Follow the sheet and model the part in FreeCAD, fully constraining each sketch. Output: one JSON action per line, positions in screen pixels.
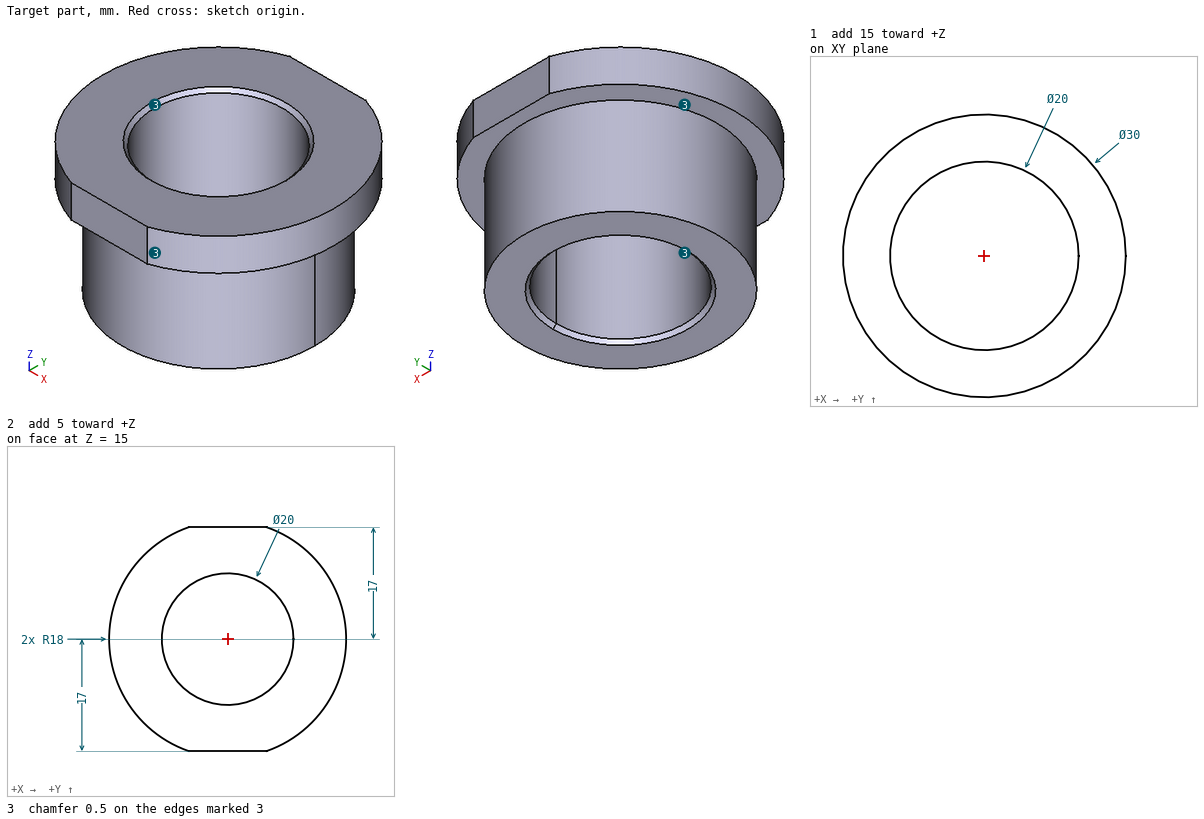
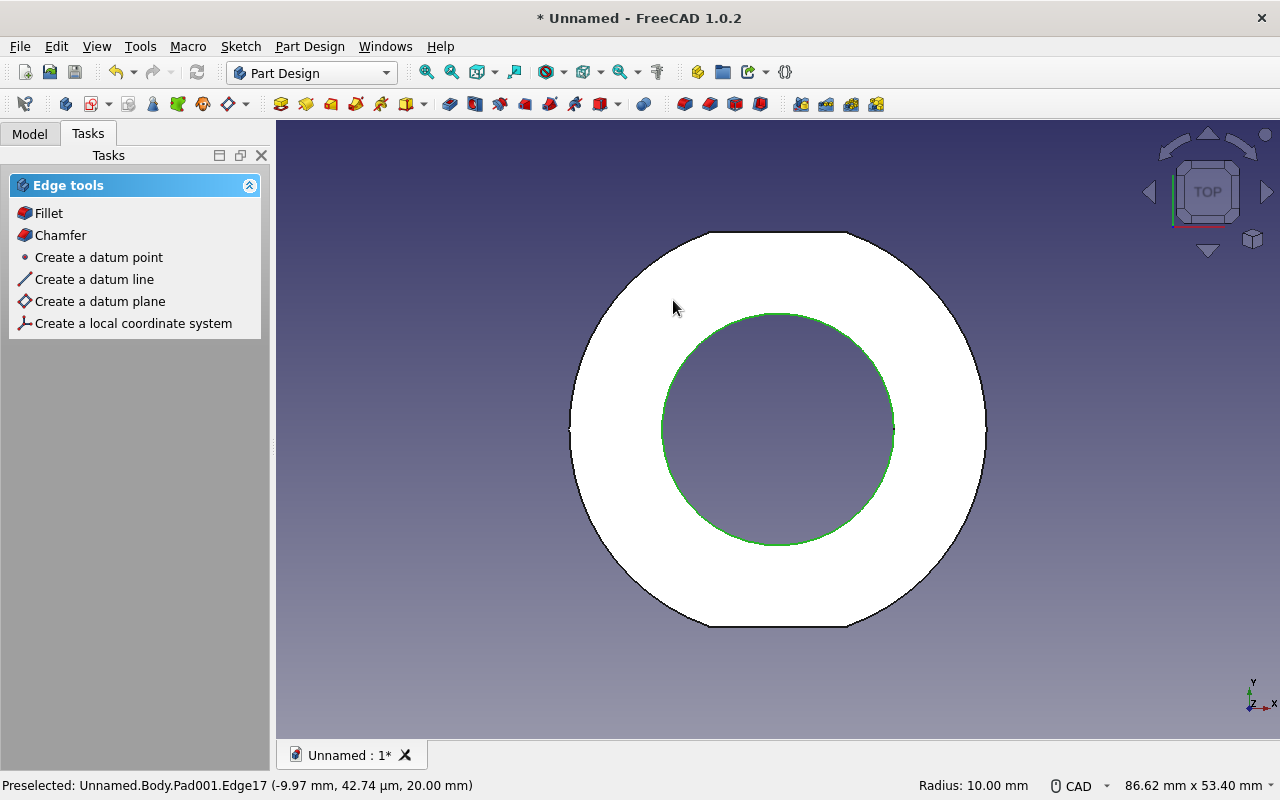
{"action": "key", "text": "1"}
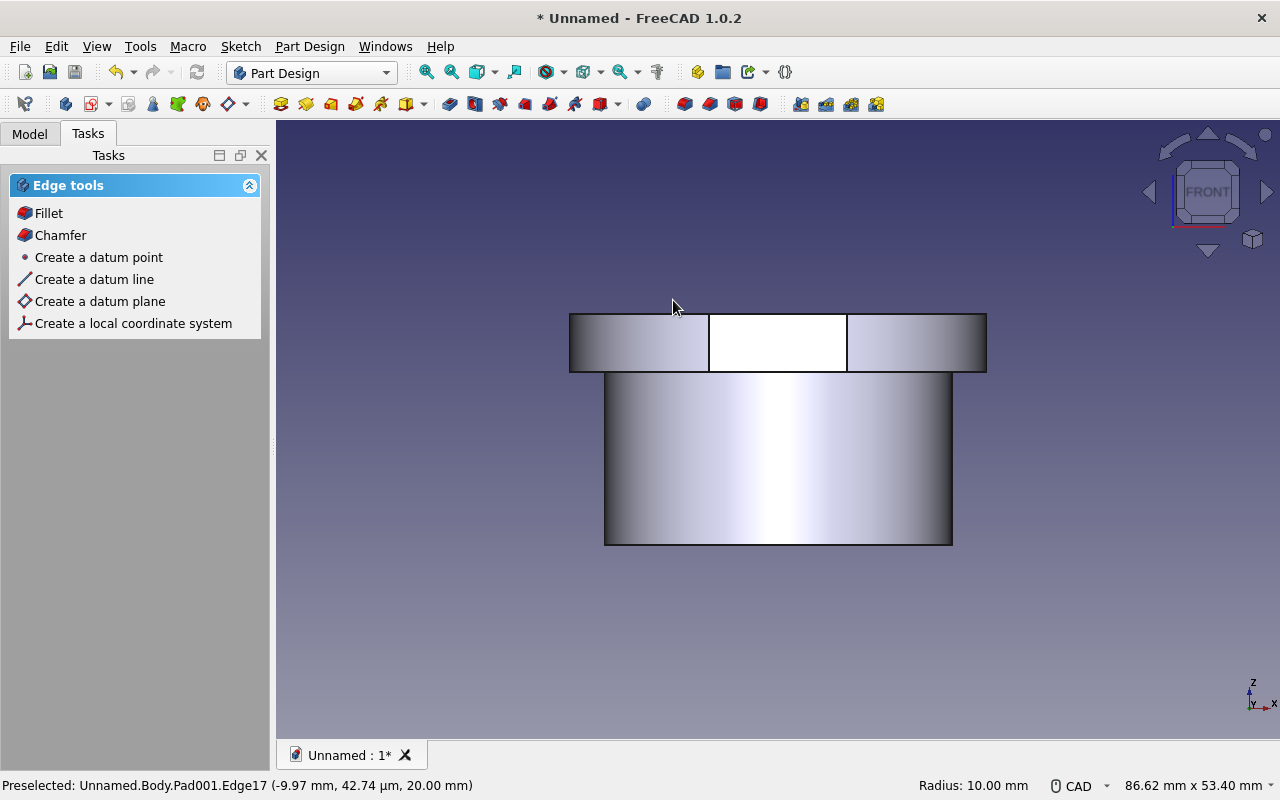
{"action": "left_click", "coordinate": [427, 72]}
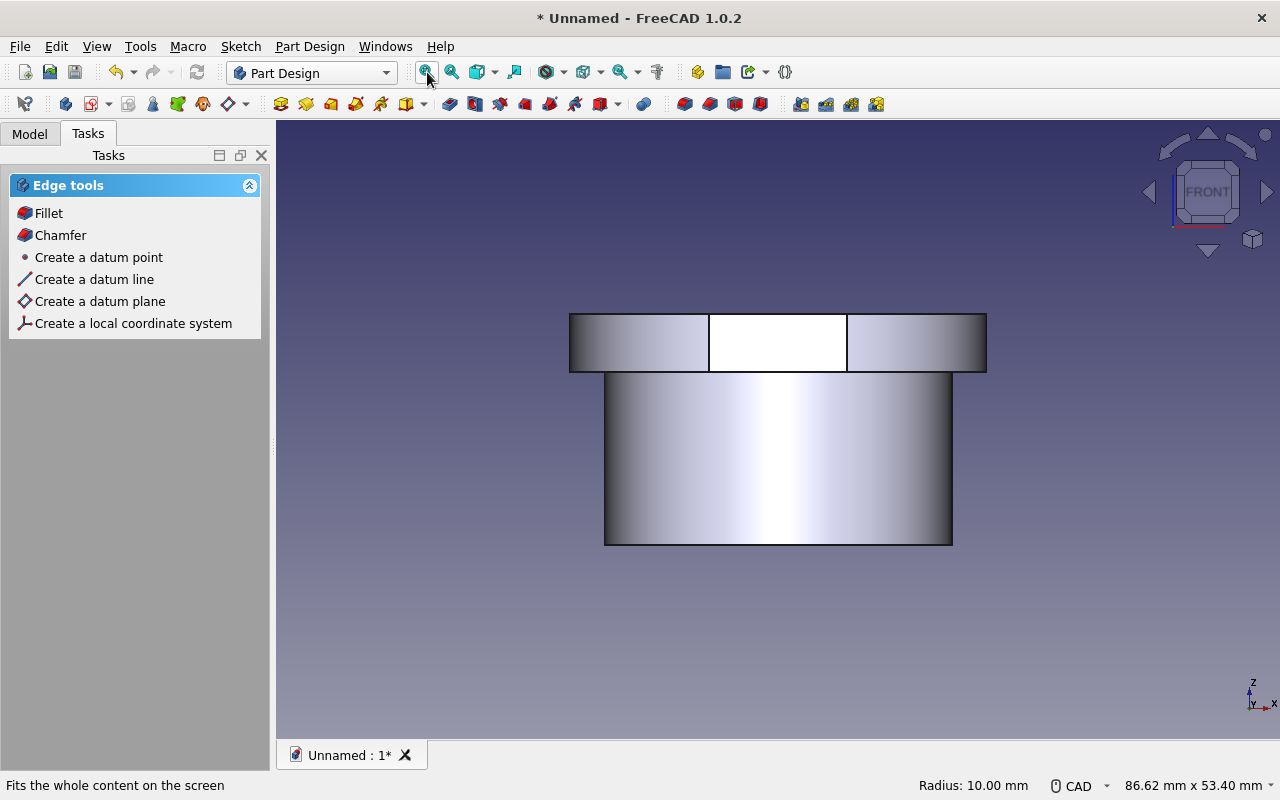
{"action": "key", "text": "3"}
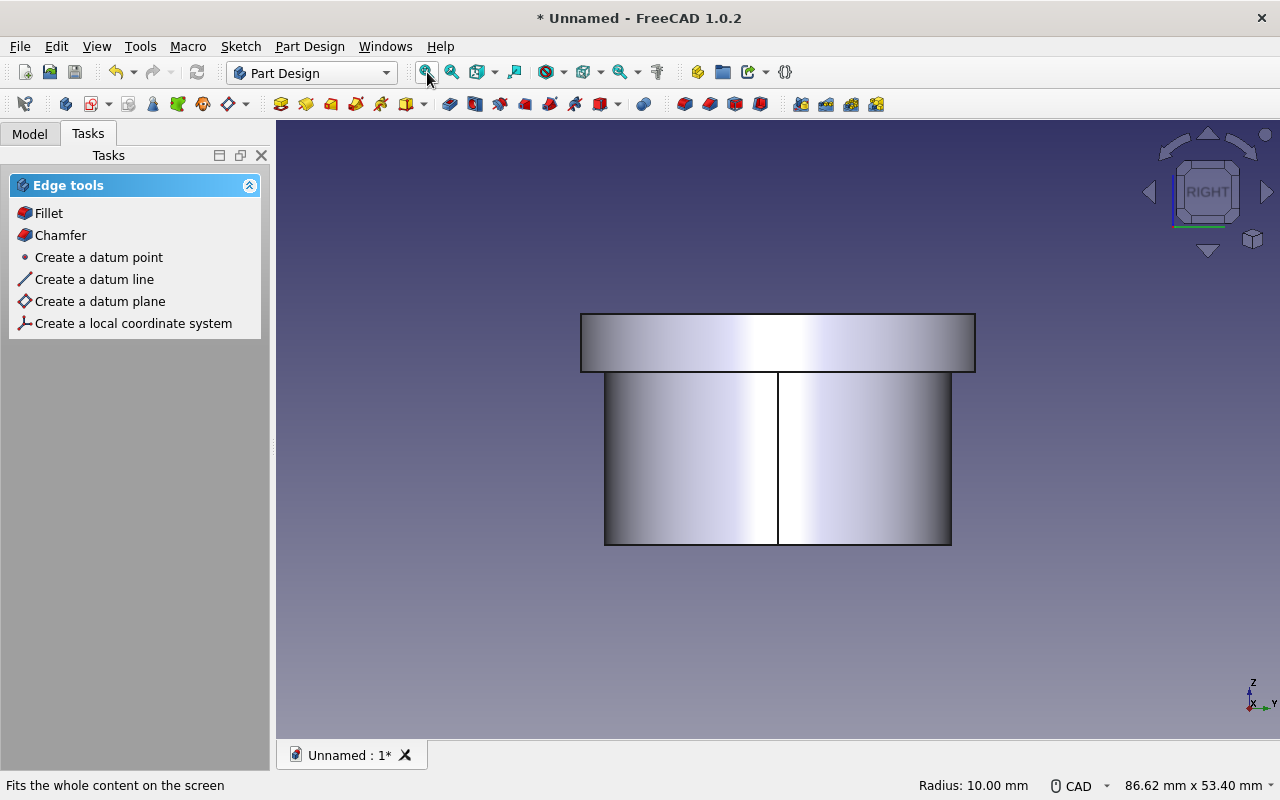
{"action": "left_click", "coordinate": [427, 72]}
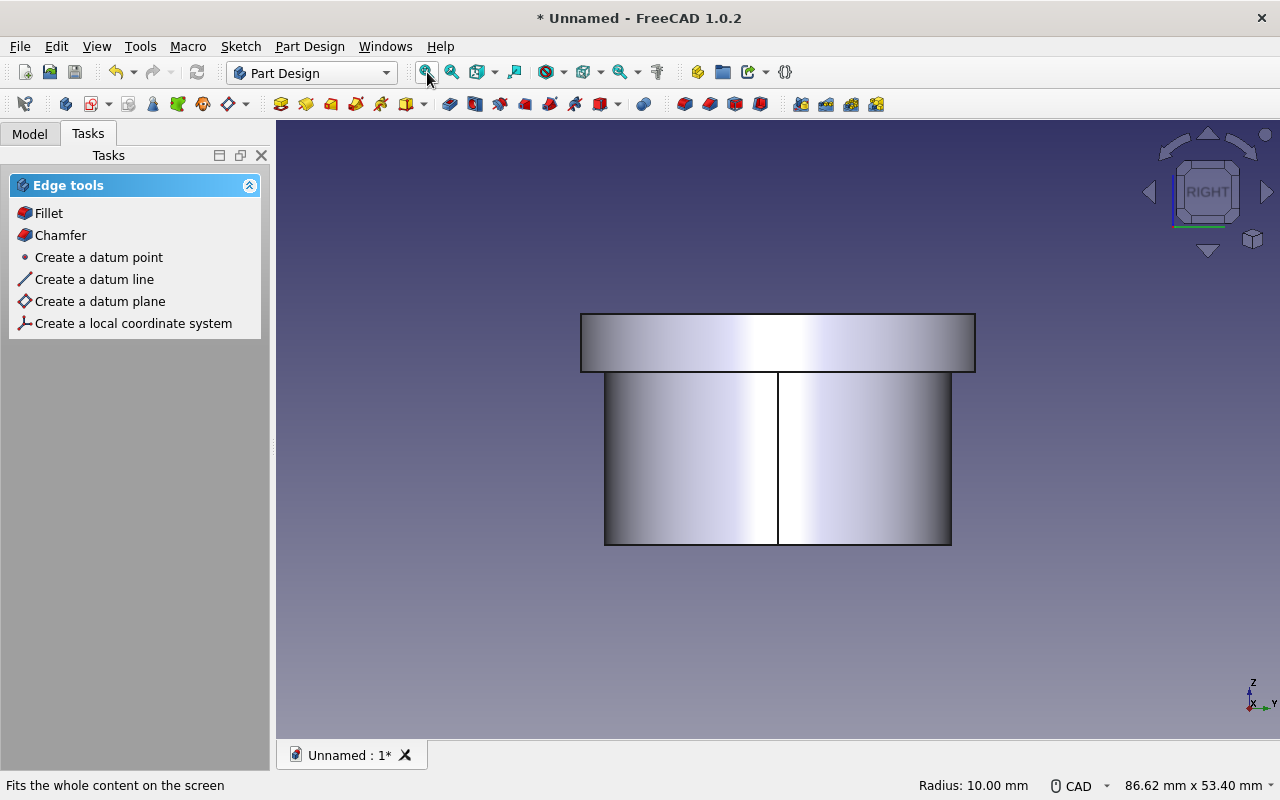
{"action": "key", "text": "5"}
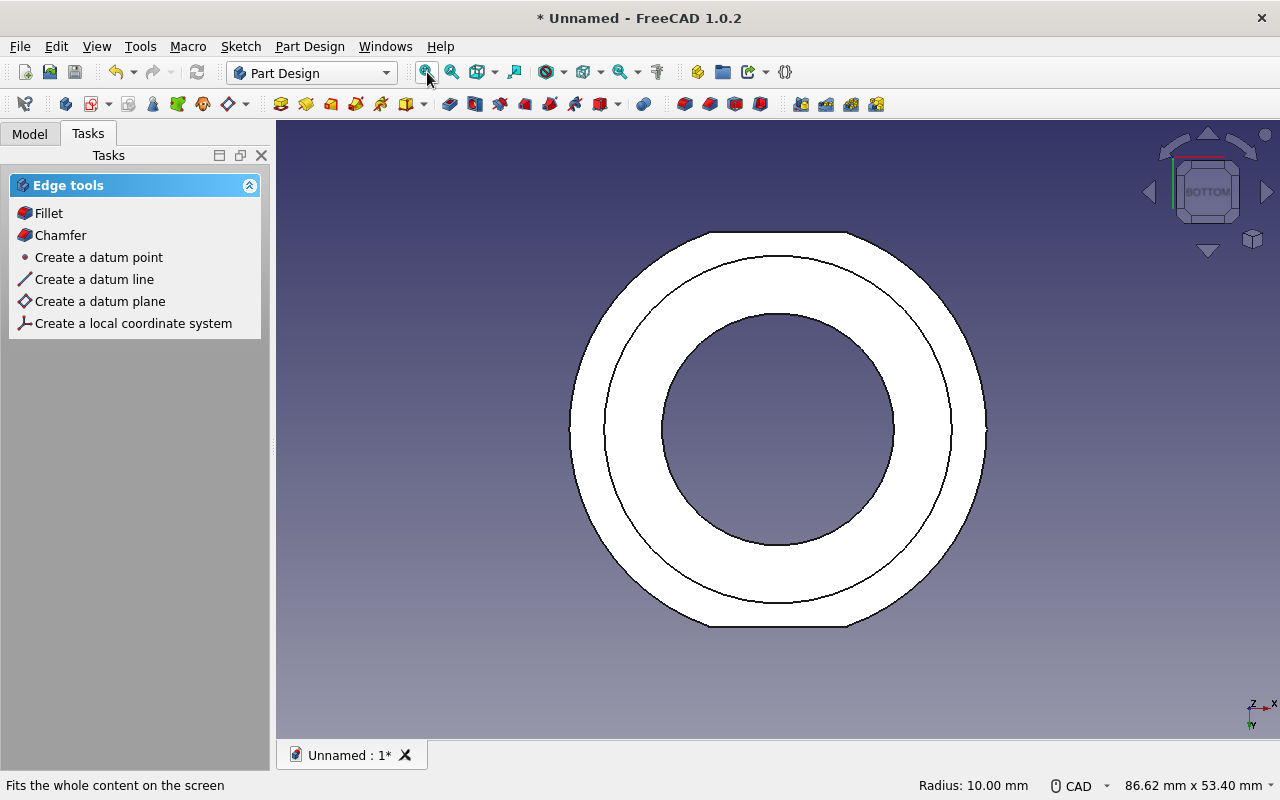
{"action": "left_click", "coordinate": [684, 497], "text": "ctrl"}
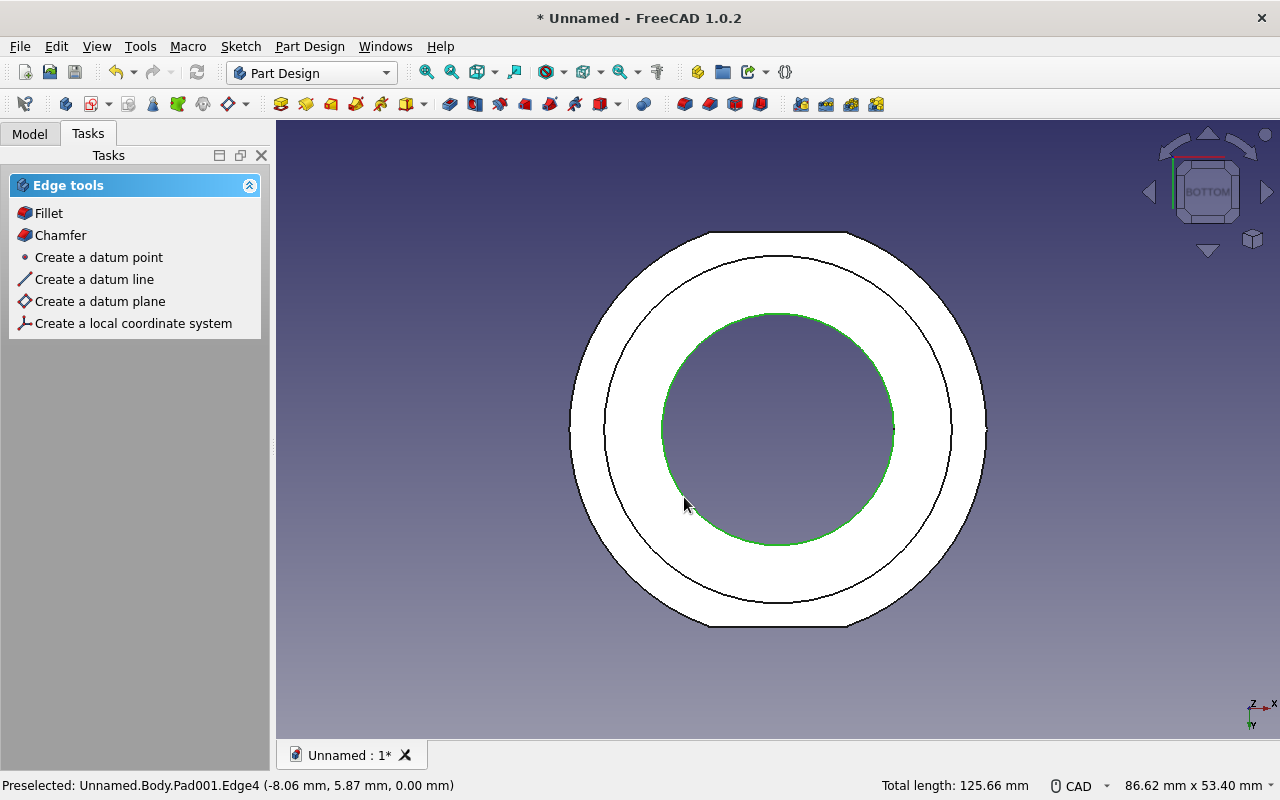
{"action": "left_click", "coordinate": [710, 104]}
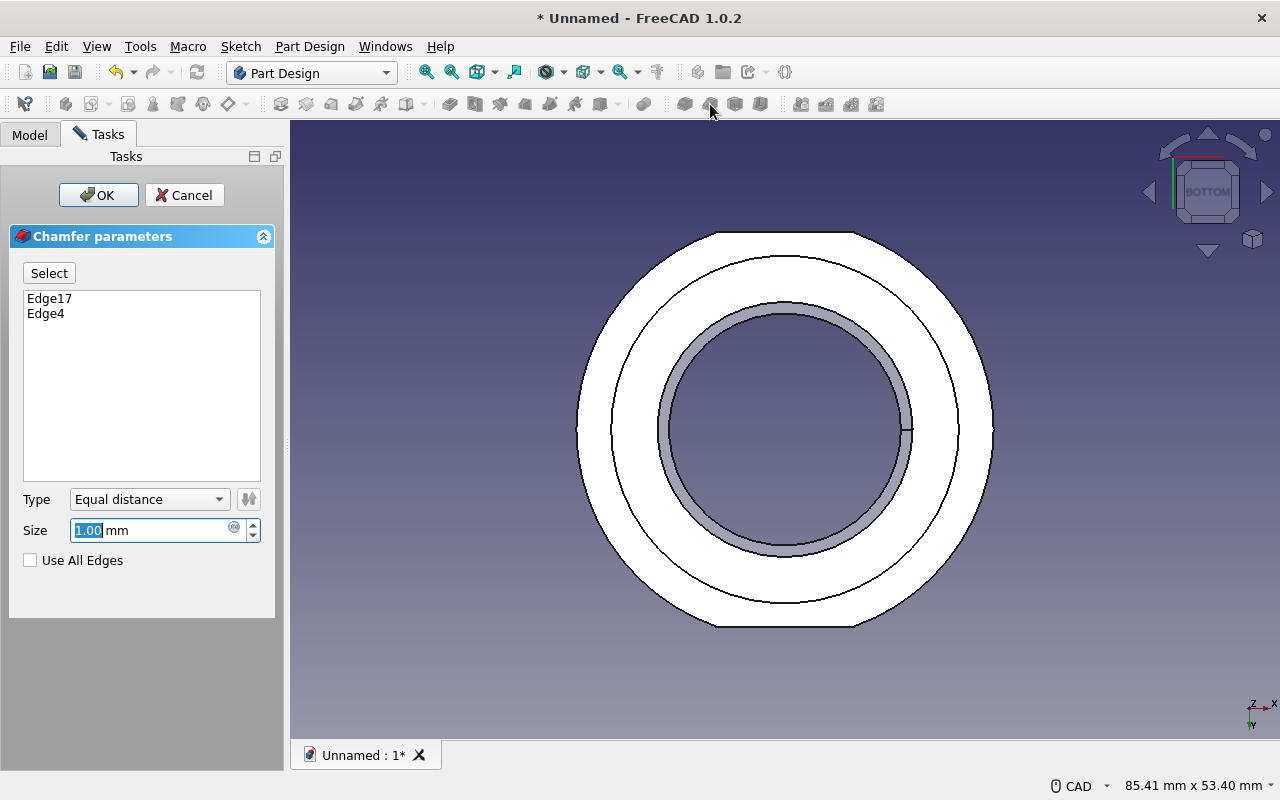
{"action": "type", "text": "0.5"}
{"action": "key", "text": "Tab"}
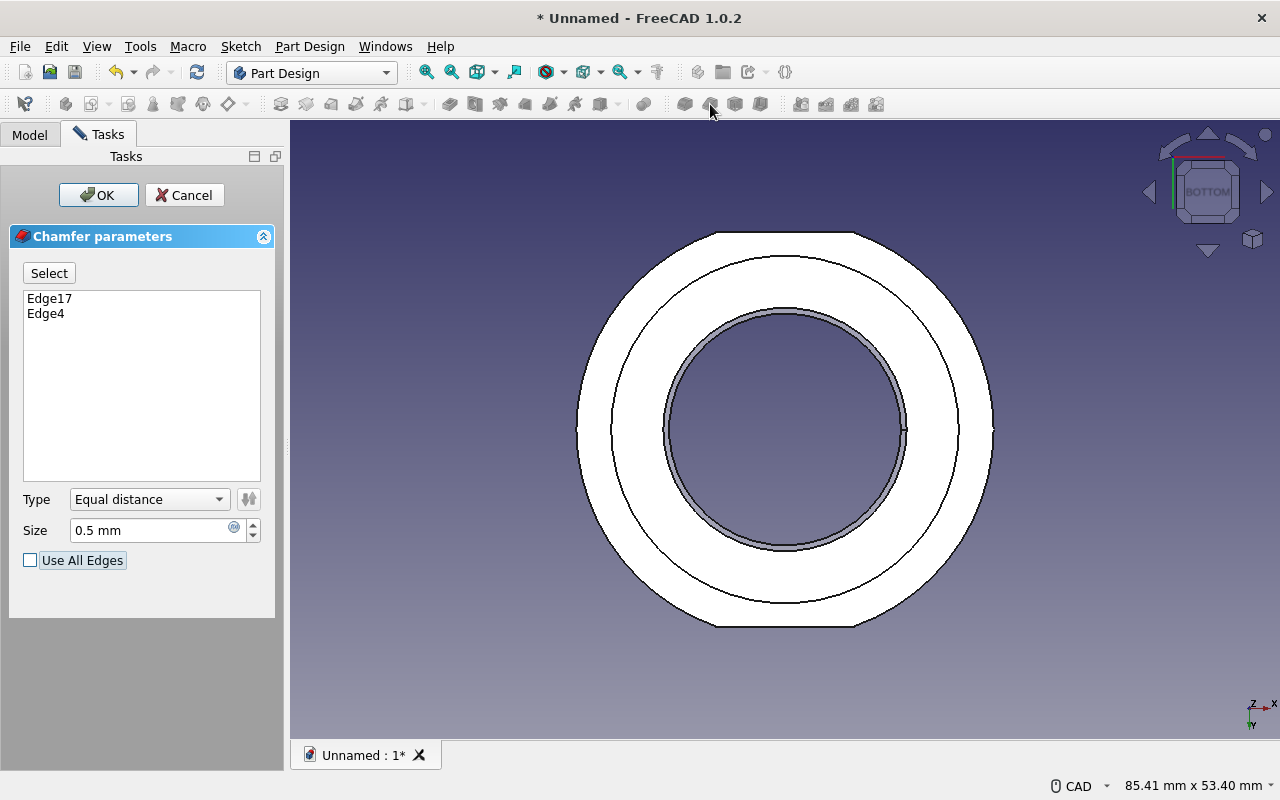
{"action": "left_click", "coordinate": [99, 195]}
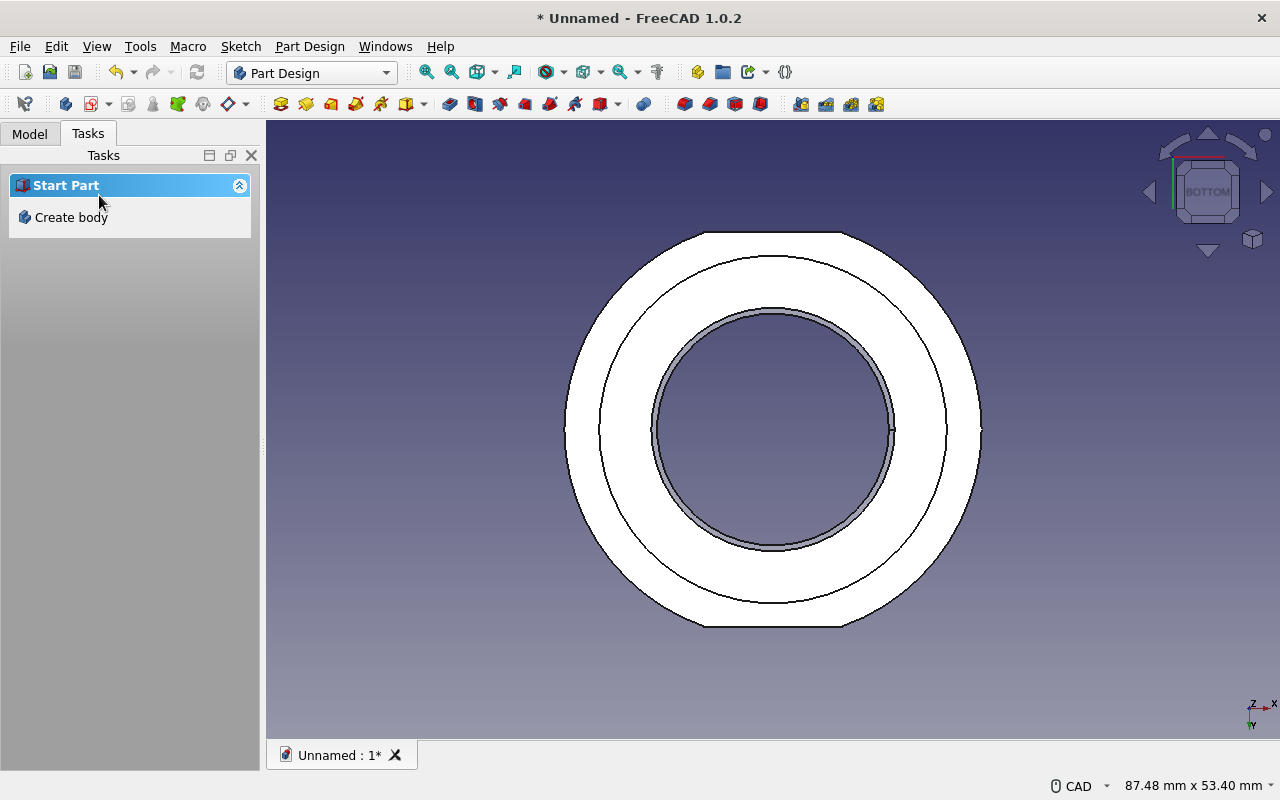
{"action": "key", "text": "0"}